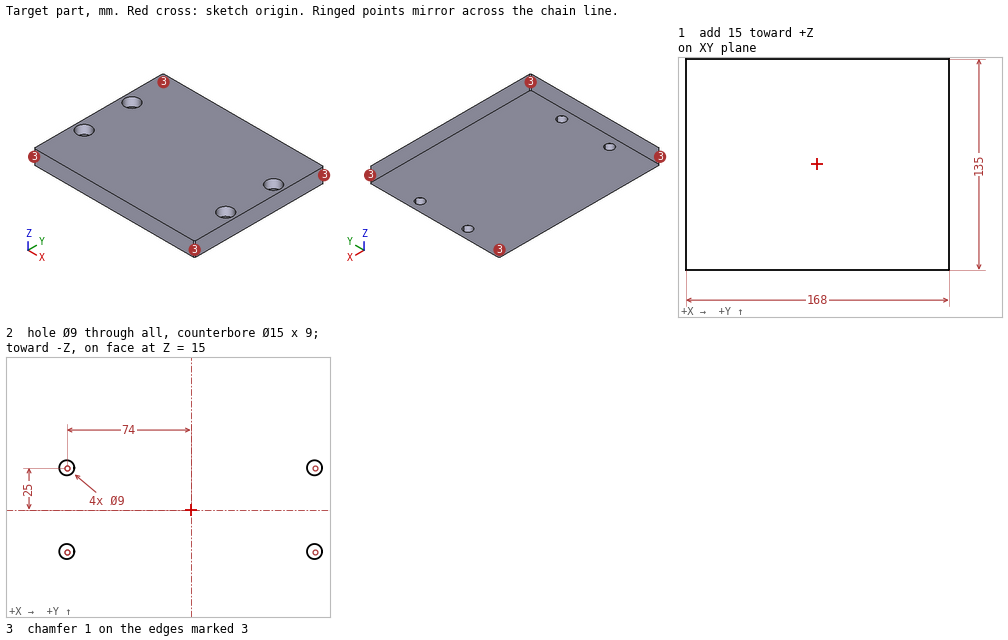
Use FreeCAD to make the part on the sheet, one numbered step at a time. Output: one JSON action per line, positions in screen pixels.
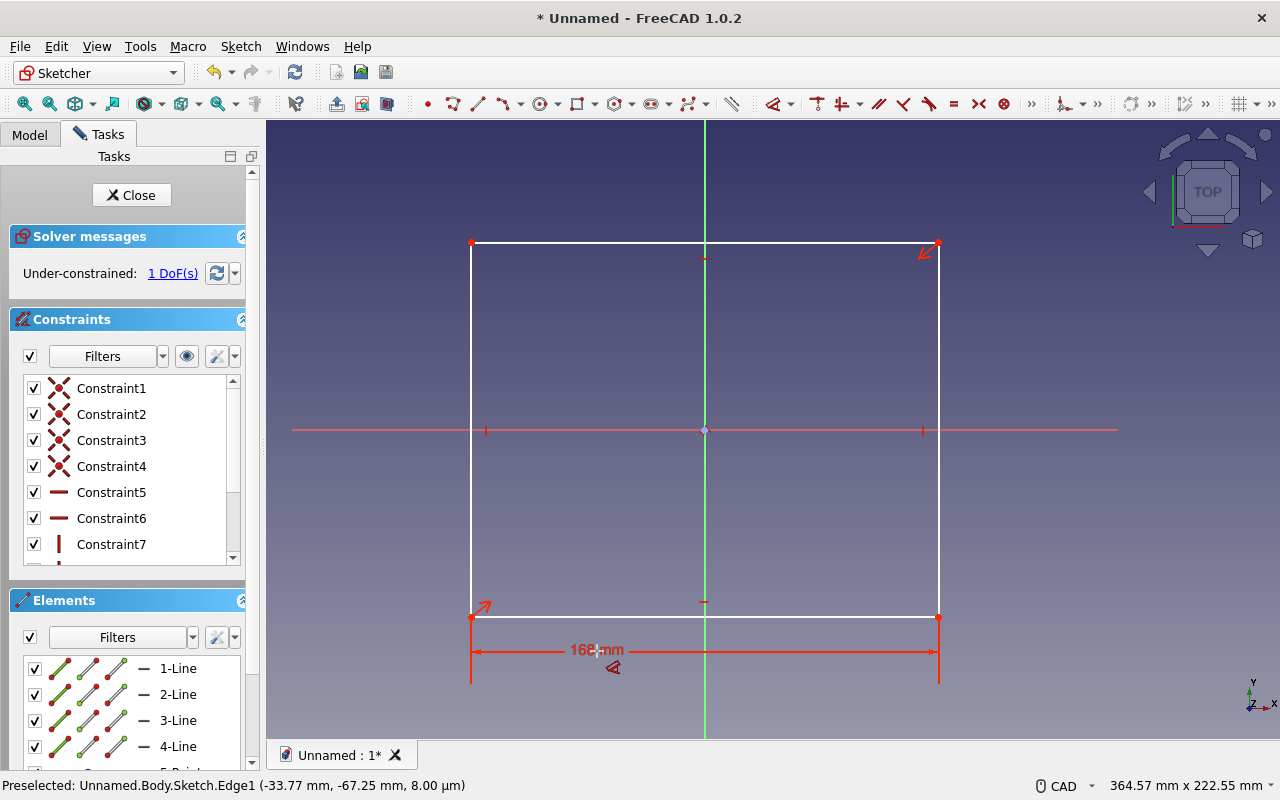
{"action": "left_click", "coordinate": [939, 505]}
{"action": "left_click", "coordinate": [973, 344]}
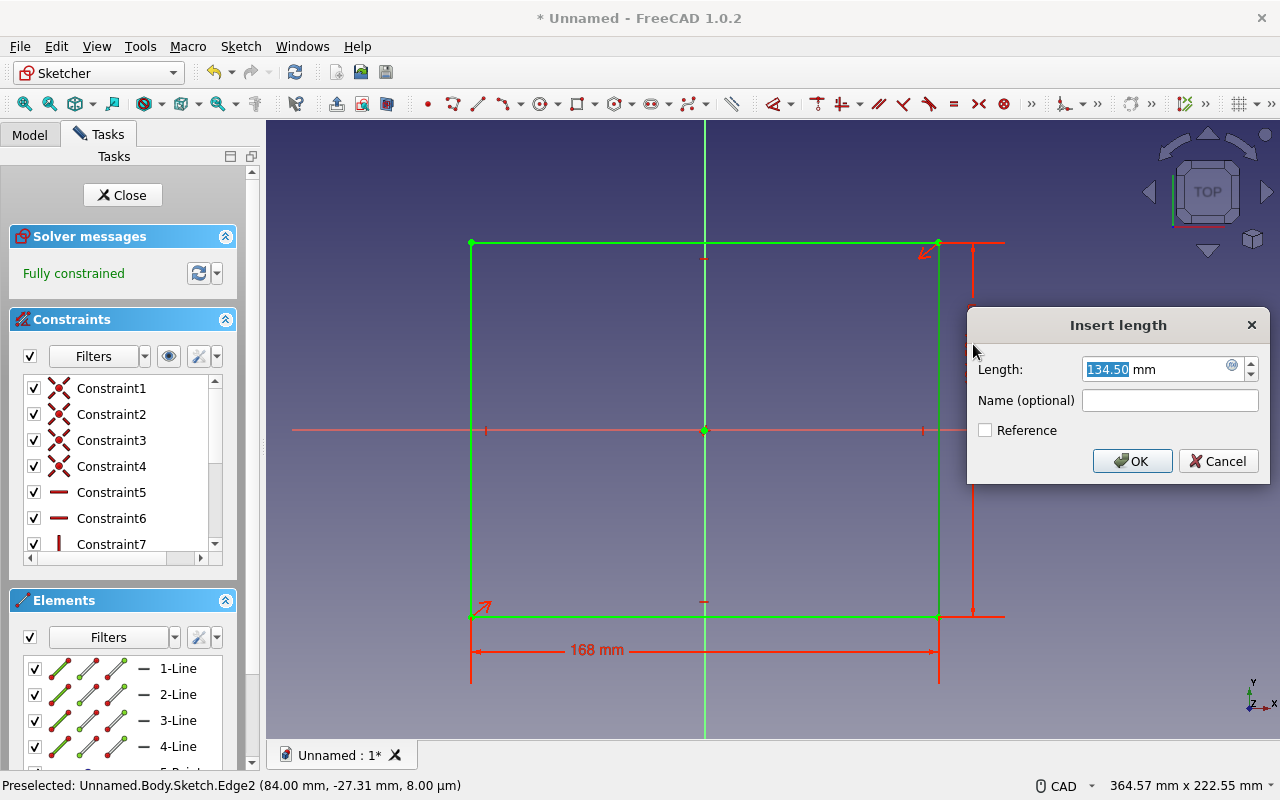
{"action": "type", "text": "135"}
{"action": "key", "text": "Return"}
{"action": "key", "text": "Escape"}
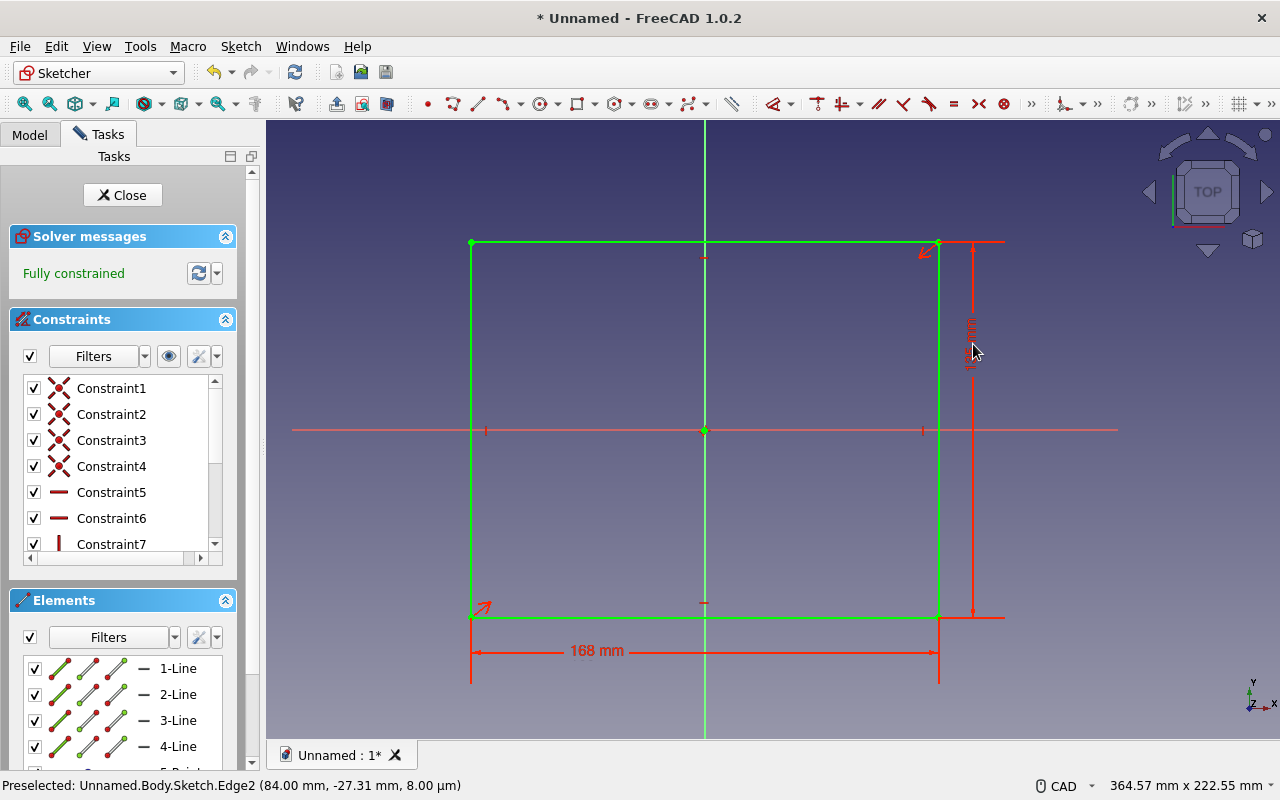
{"action": "left_click", "coordinate": [123, 195]}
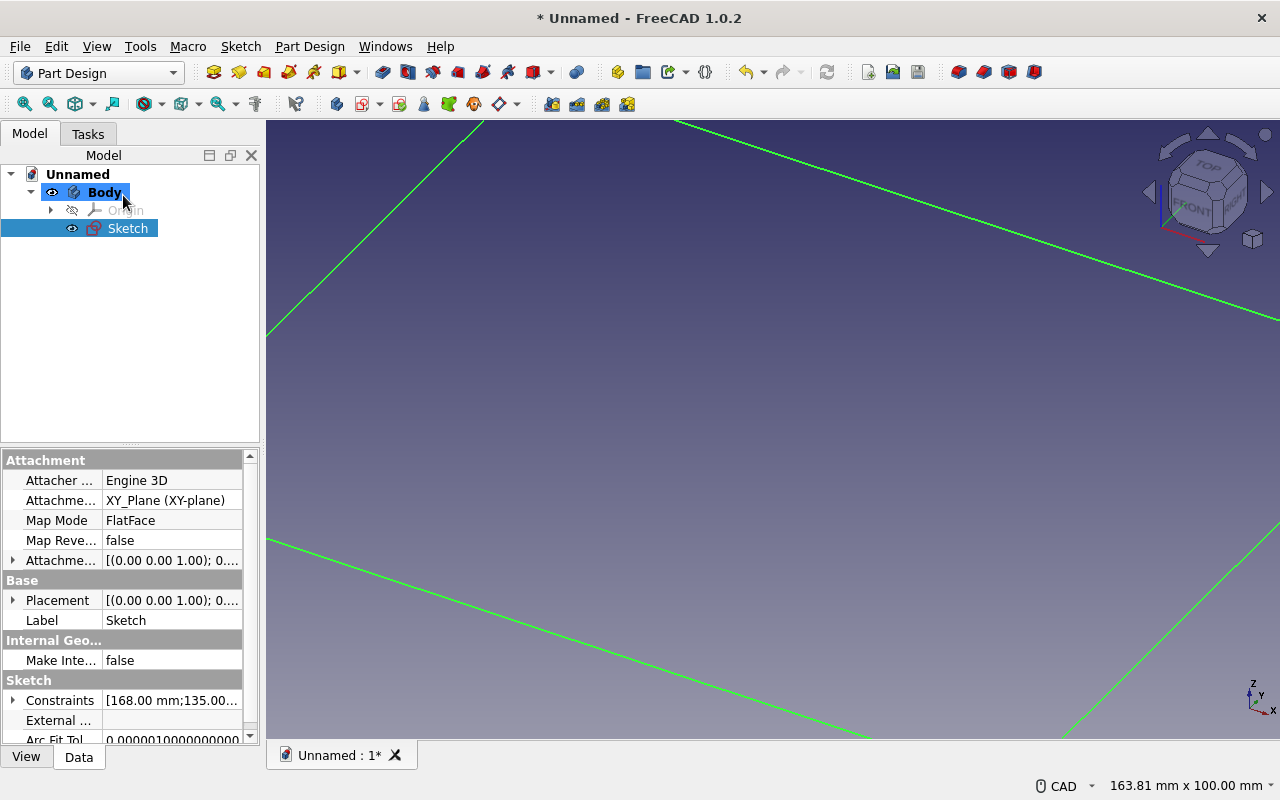
{"action": "left_click", "coordinate": [214, 72]}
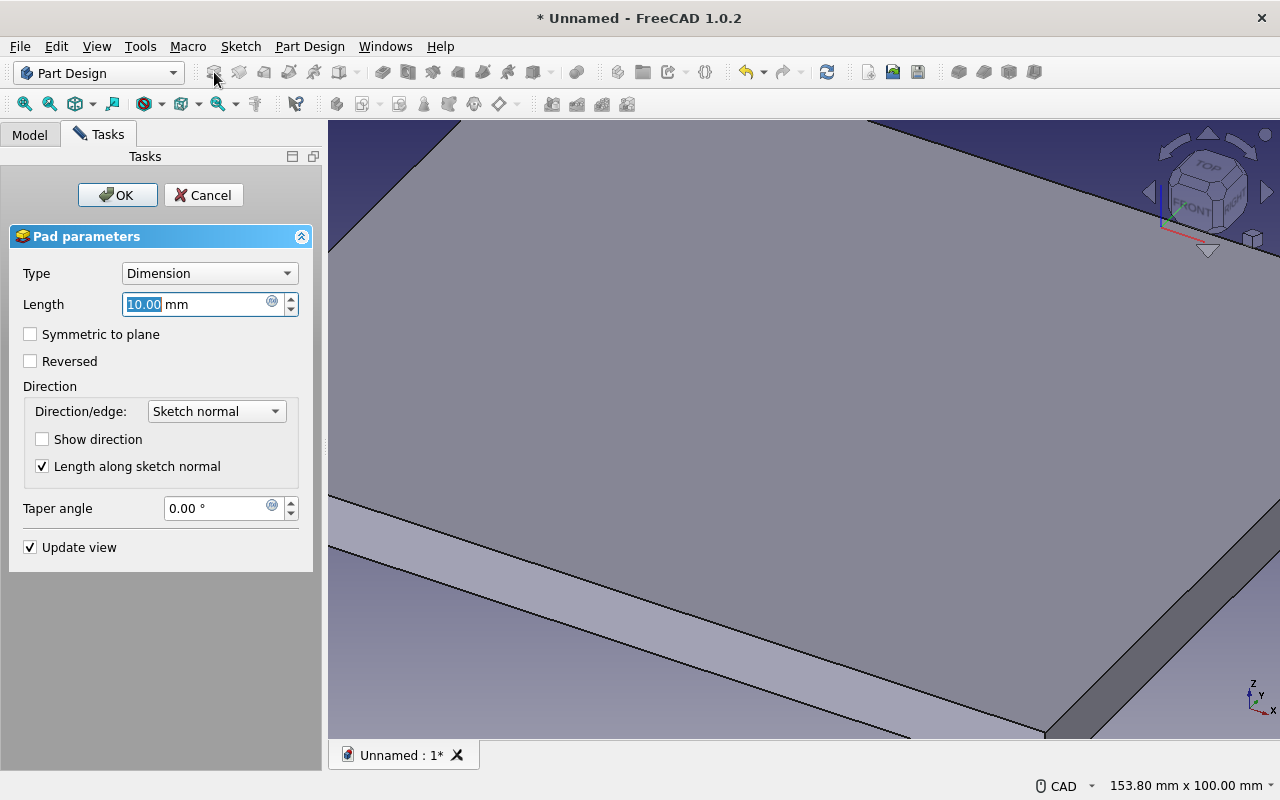
{"action": "type", "text": "15"}
{"action": "key", "text": "Tab"}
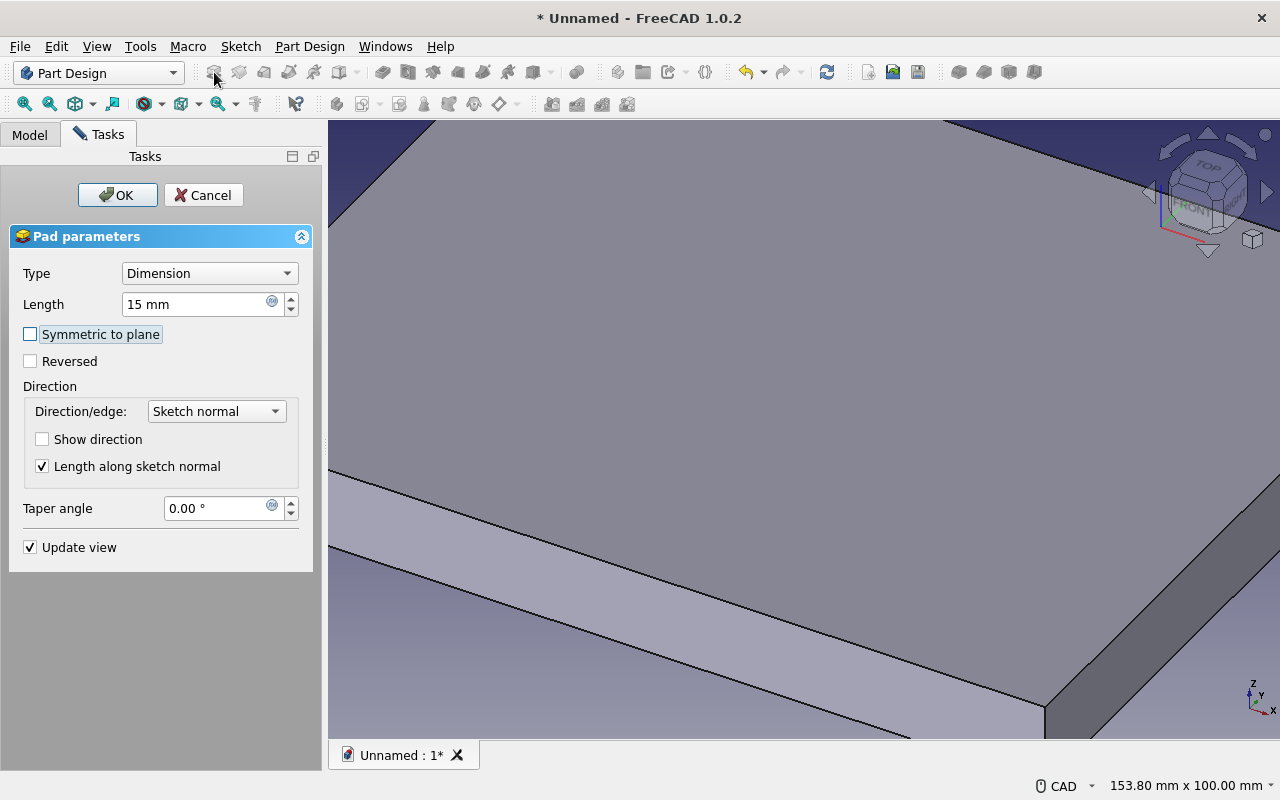
{"action": "left_click", "coordinate": [118, 195]}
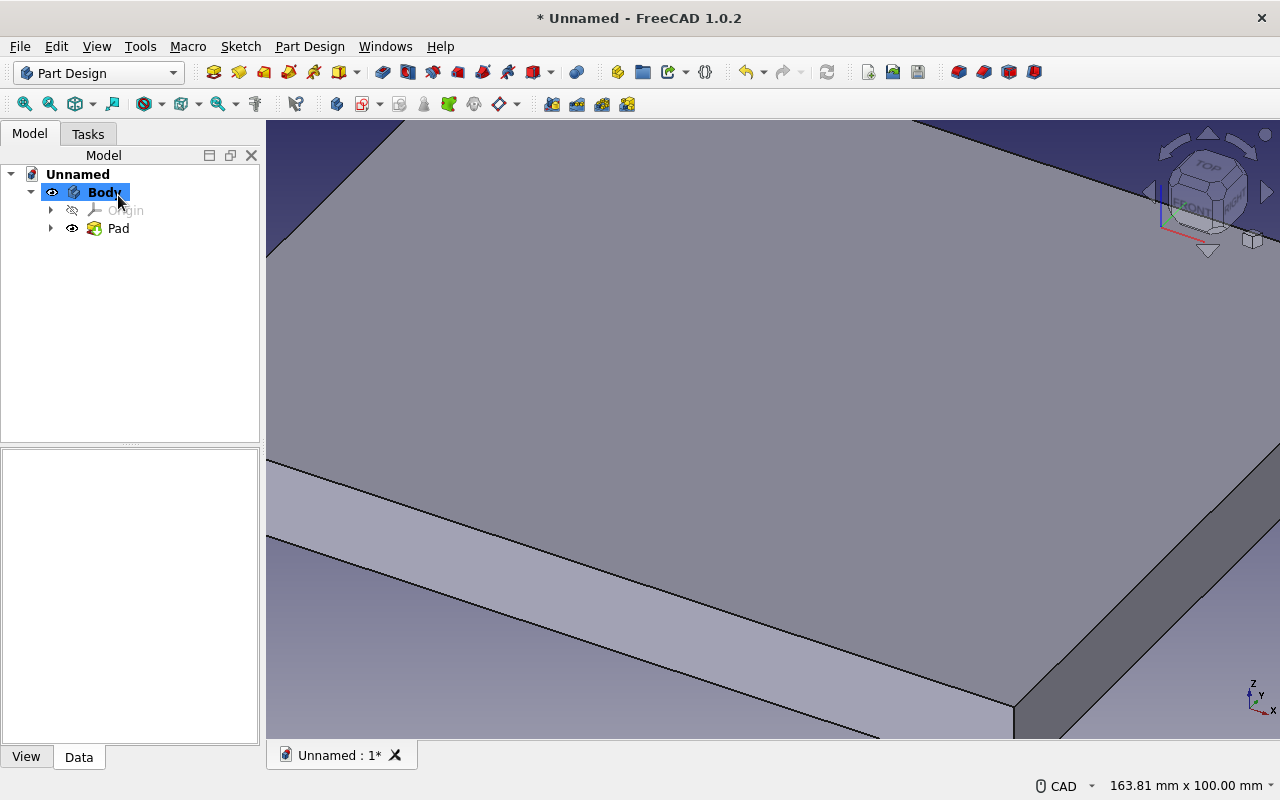
{"action": "key", "text": "v f"}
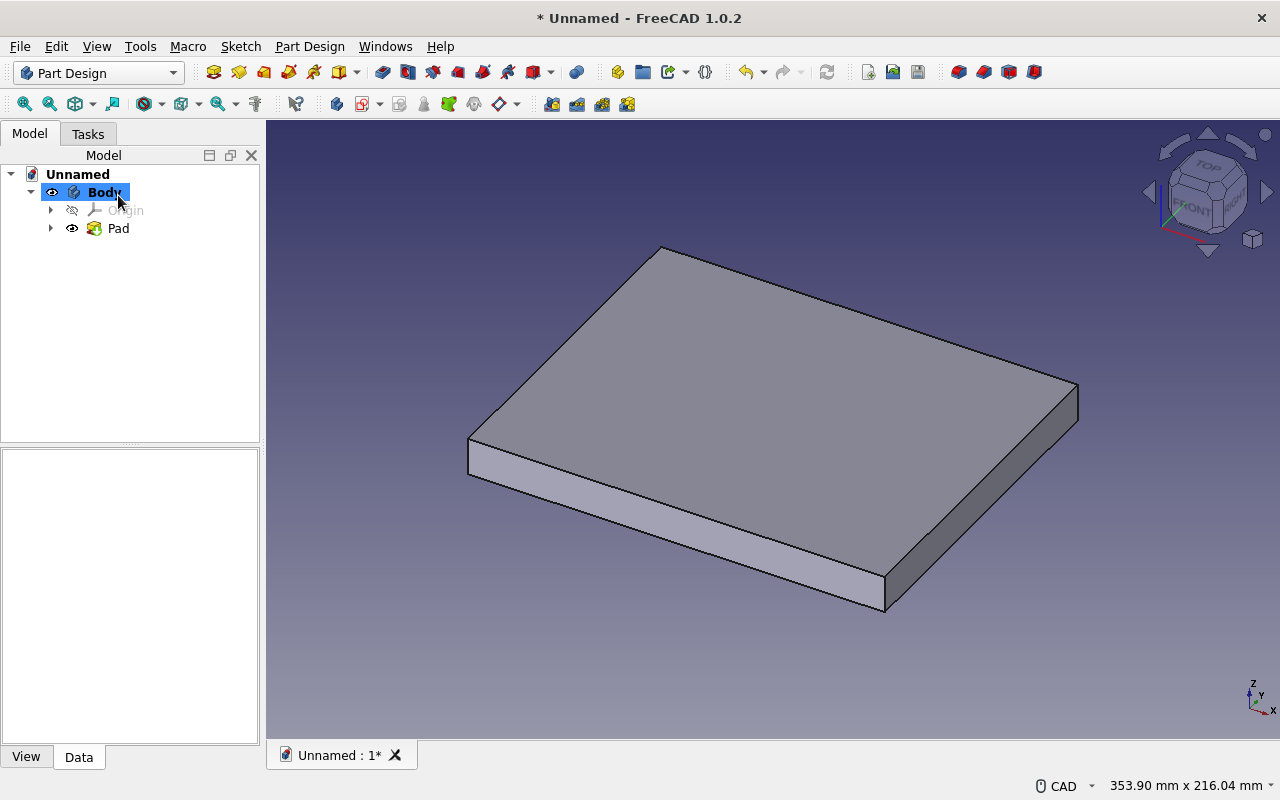
{"action": "left_click", "coordinate": [773, 411]}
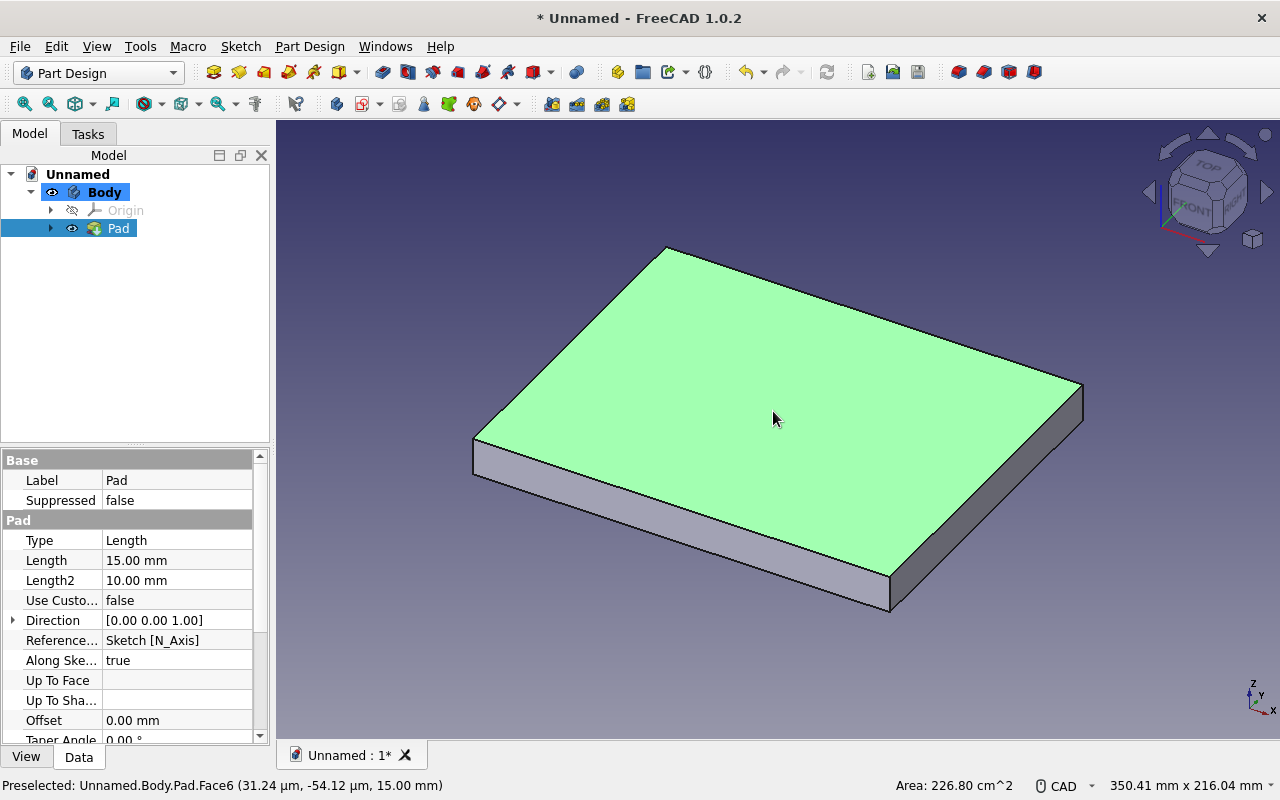
{"action": "left_click", "coordinate": [362, 104]}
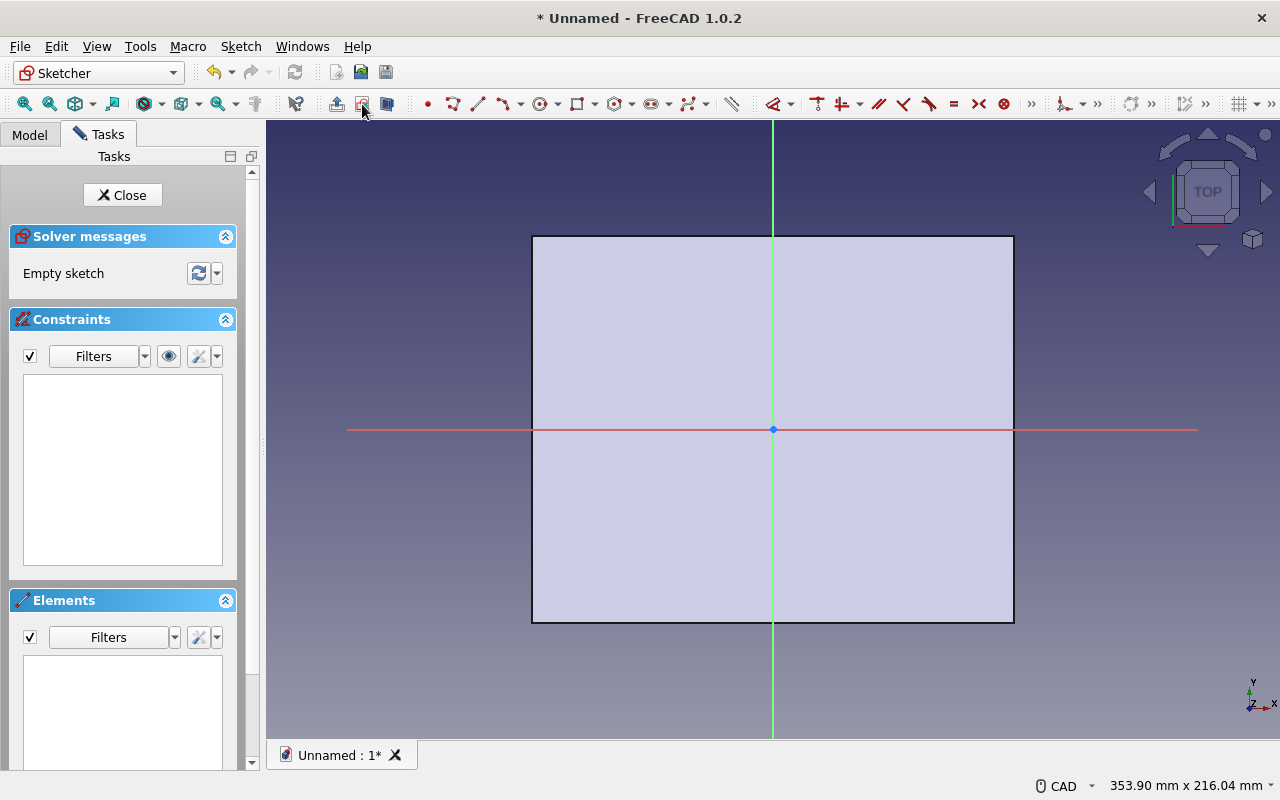
{"action": "left_click", "coordinate": [540, 104]}